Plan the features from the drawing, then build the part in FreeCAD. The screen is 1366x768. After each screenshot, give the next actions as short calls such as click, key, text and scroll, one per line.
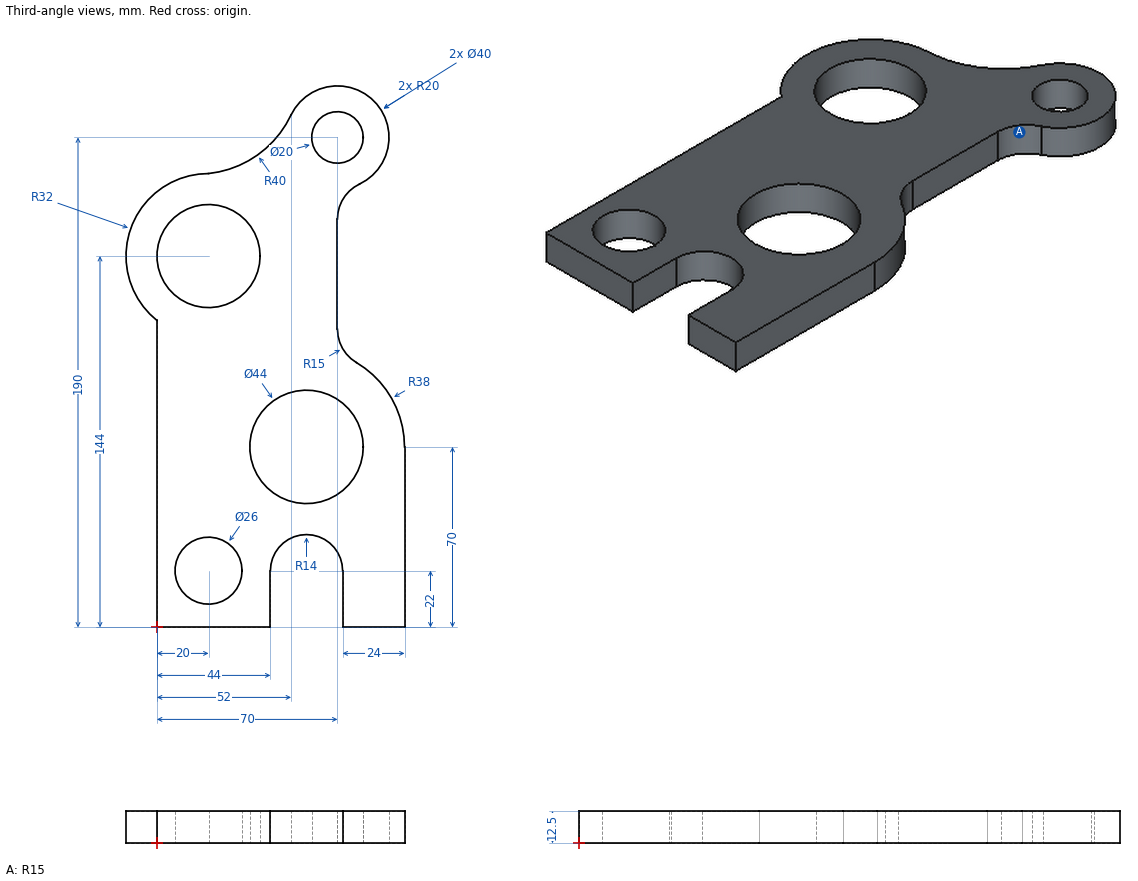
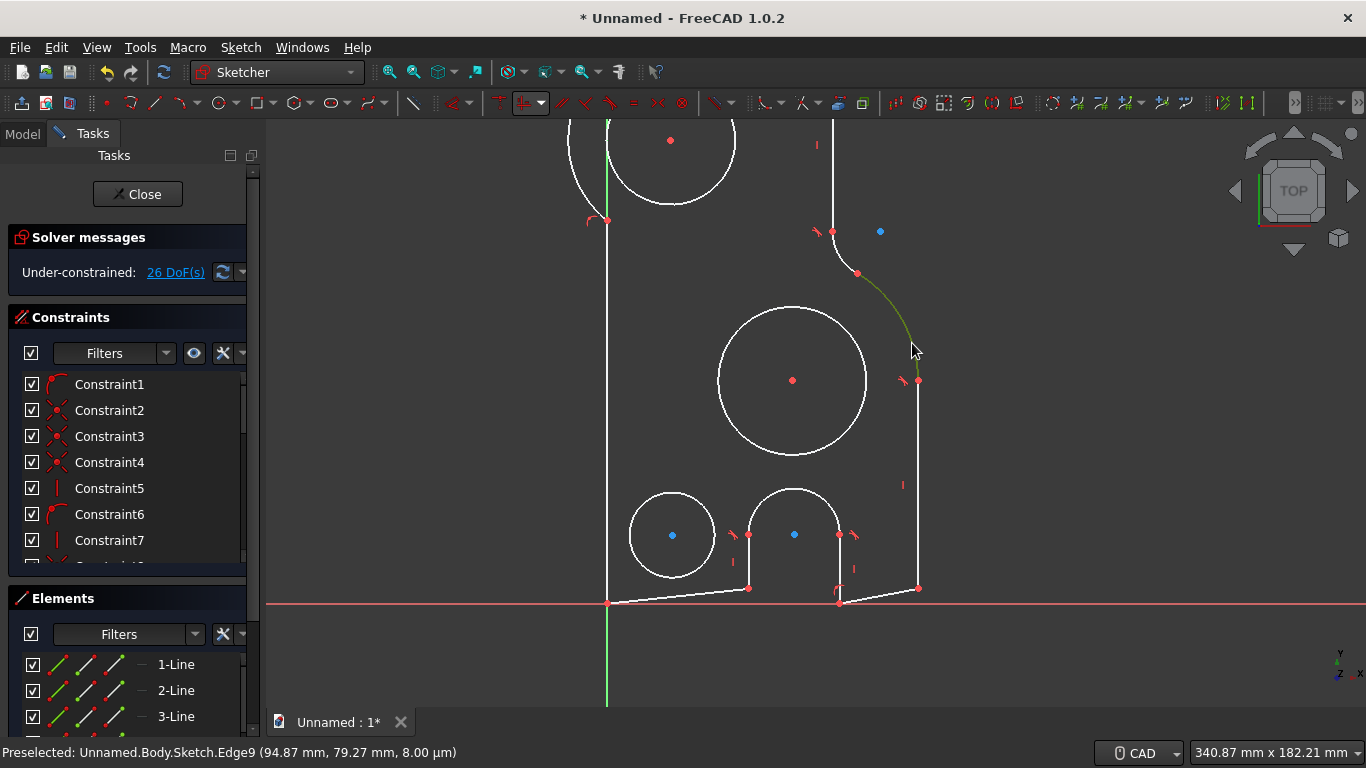
click(835, 247)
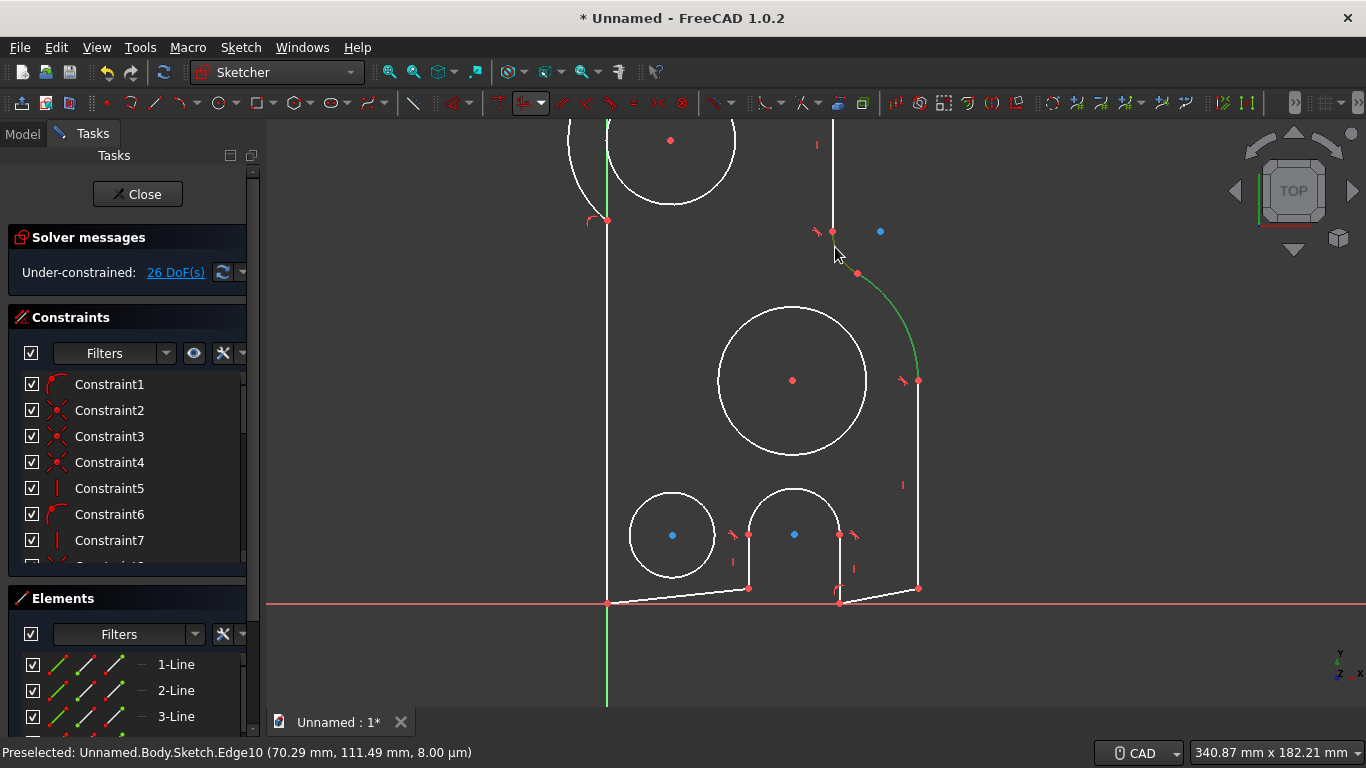
click(610, 104)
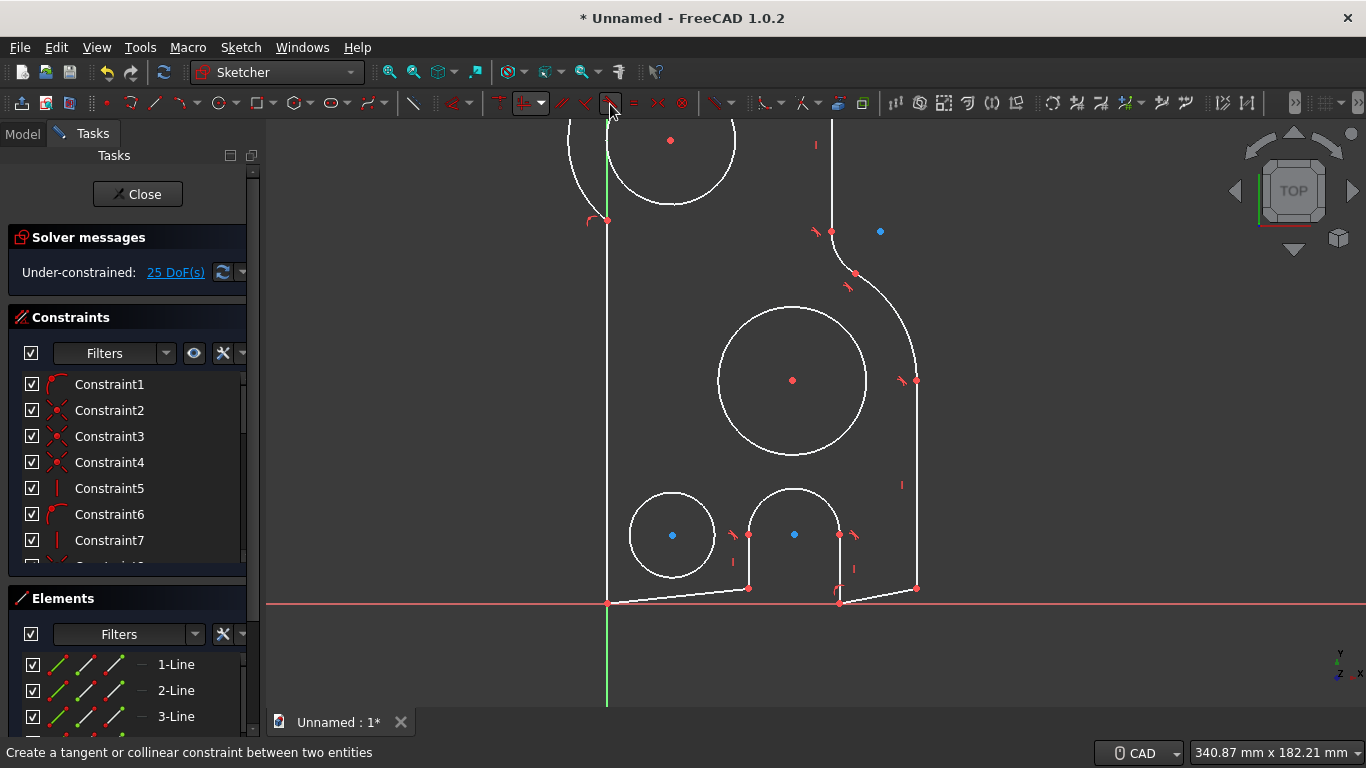
scroll(706, 593, up, 2)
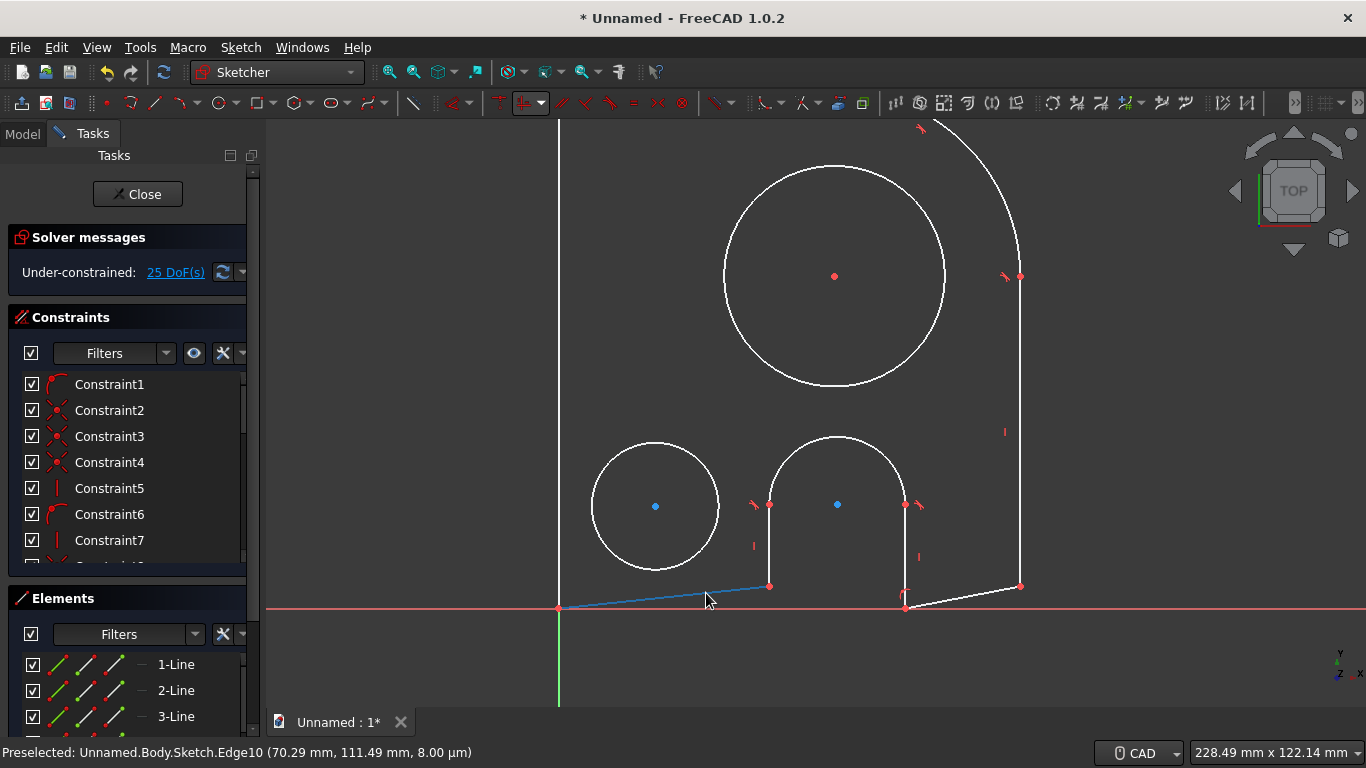
click(706, 593)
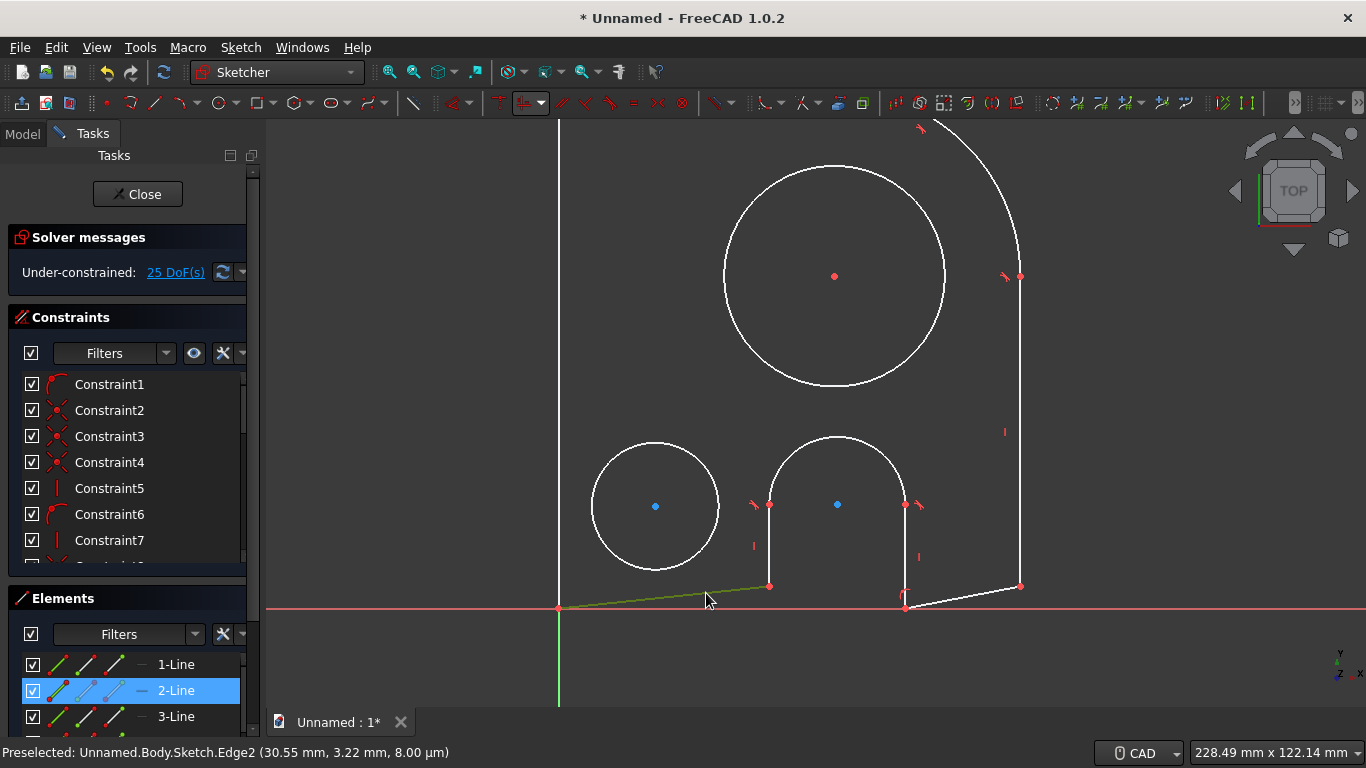
click(544, 104)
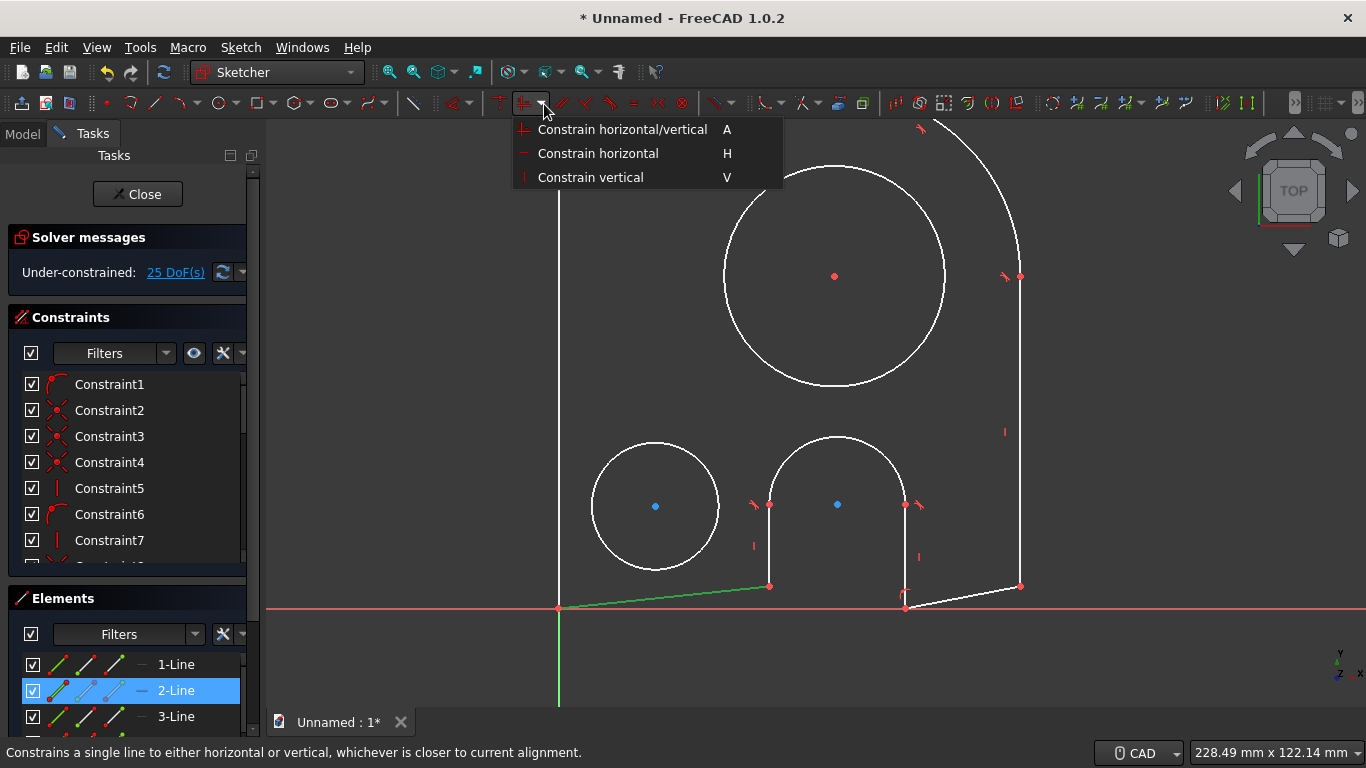
click(648, 153)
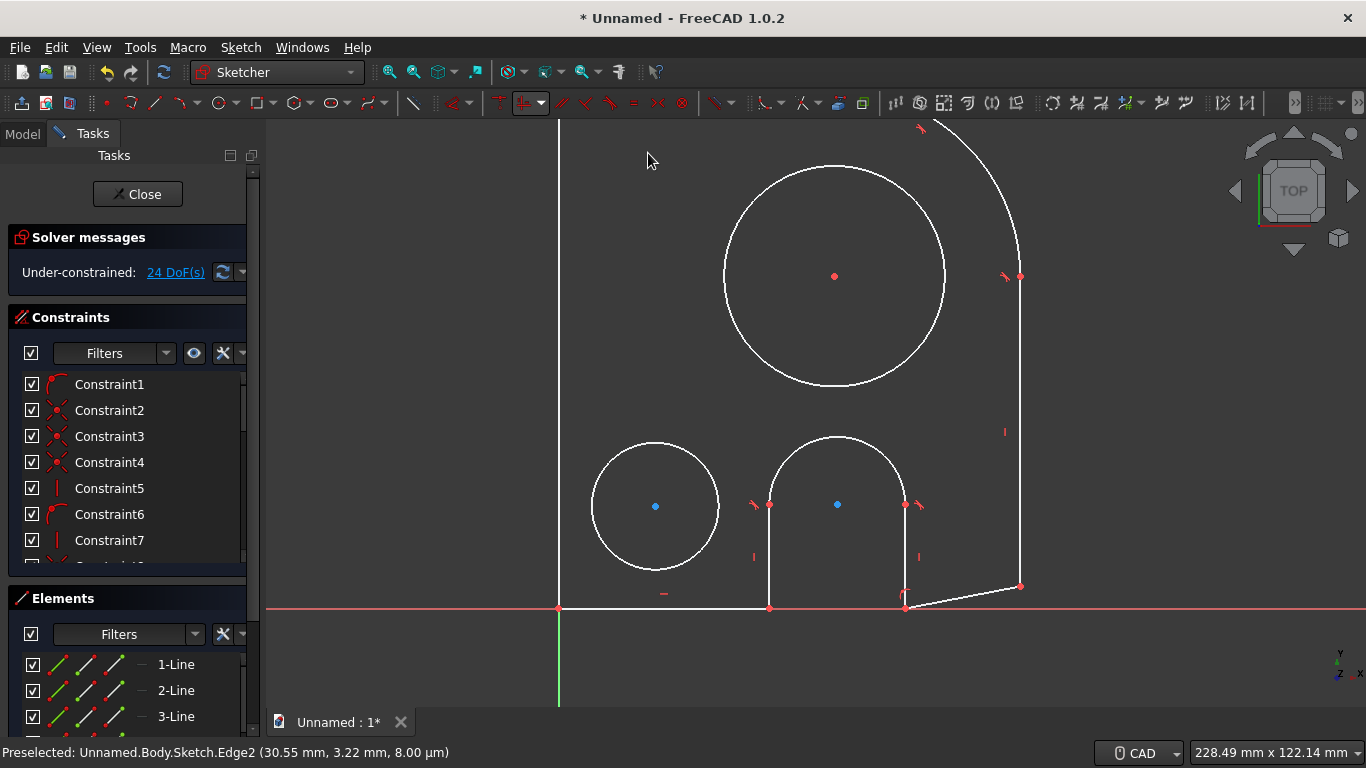
click(986, 593)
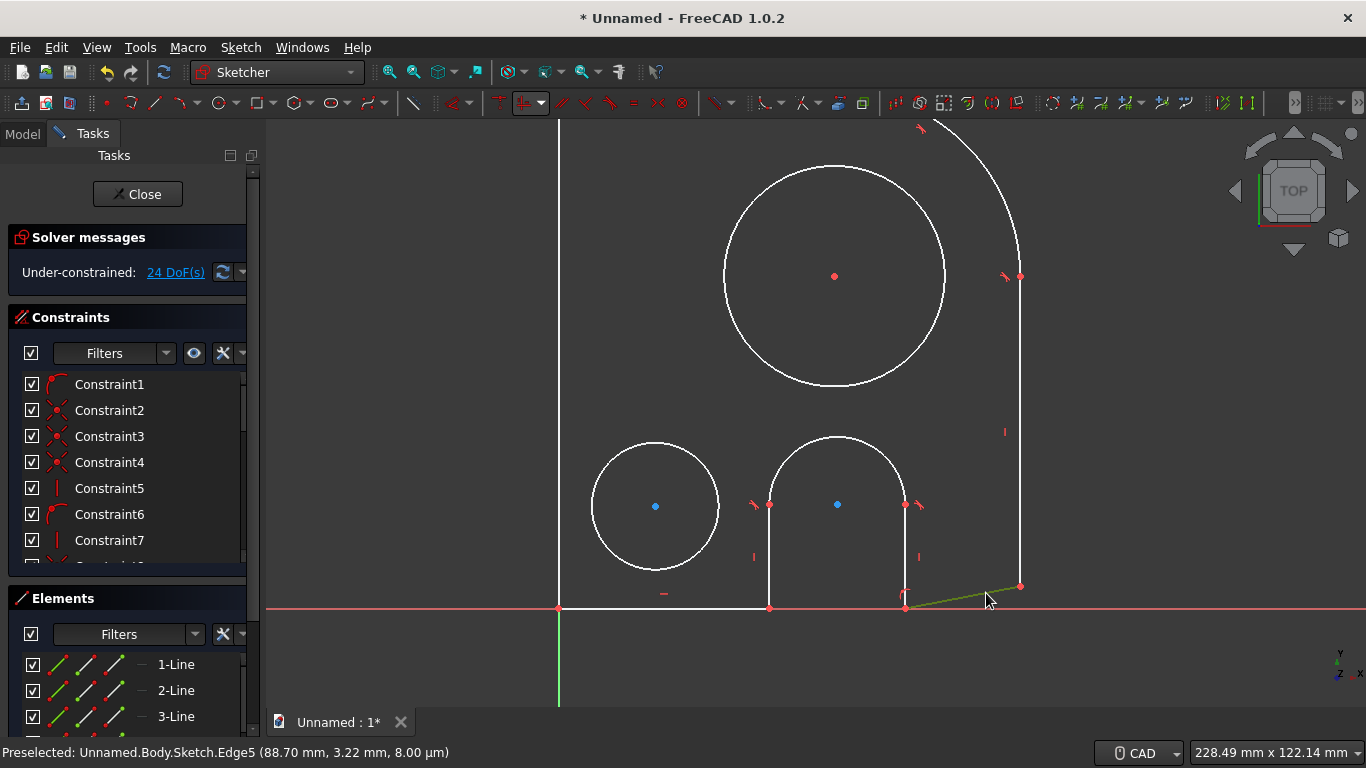
key(h)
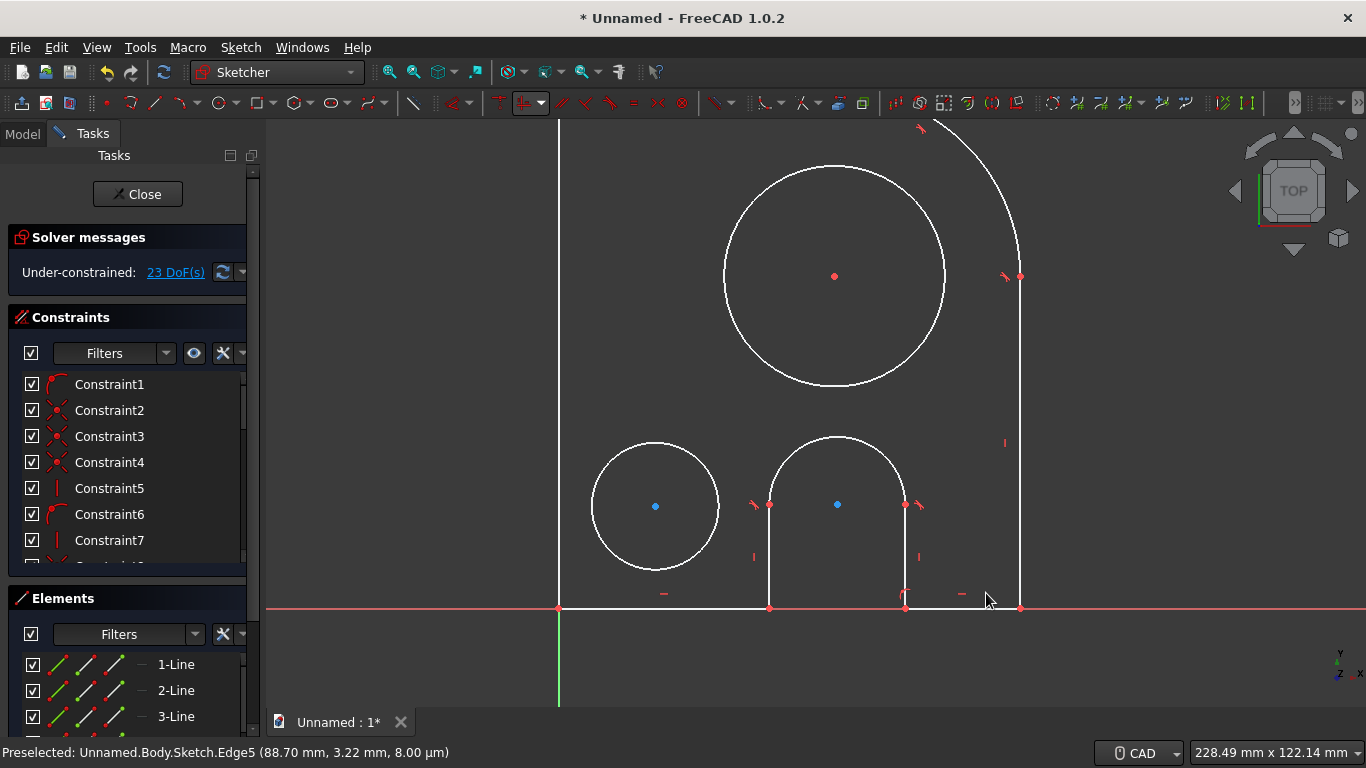
click(452, 104)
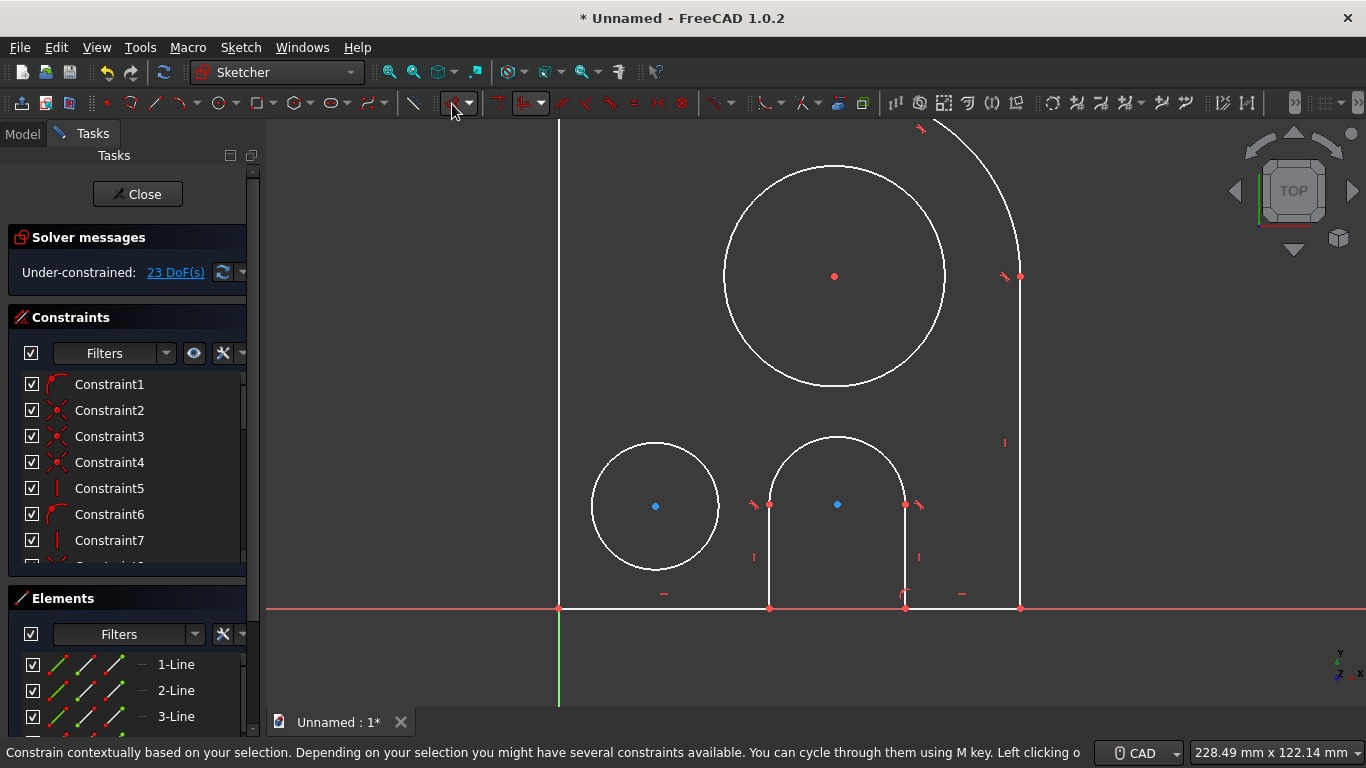
click(877, 450)
click(896, 424)